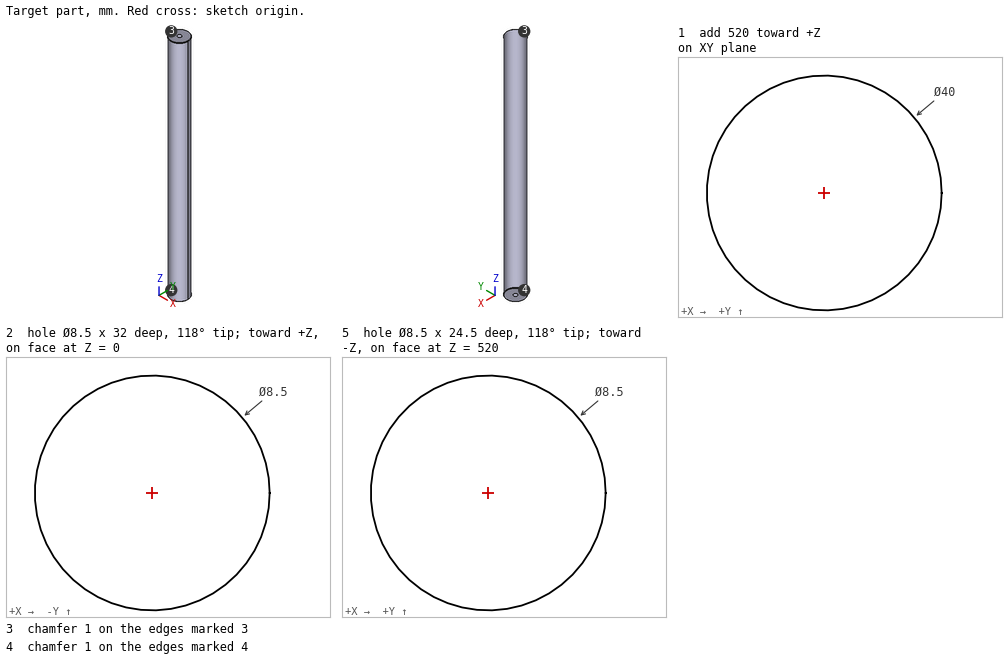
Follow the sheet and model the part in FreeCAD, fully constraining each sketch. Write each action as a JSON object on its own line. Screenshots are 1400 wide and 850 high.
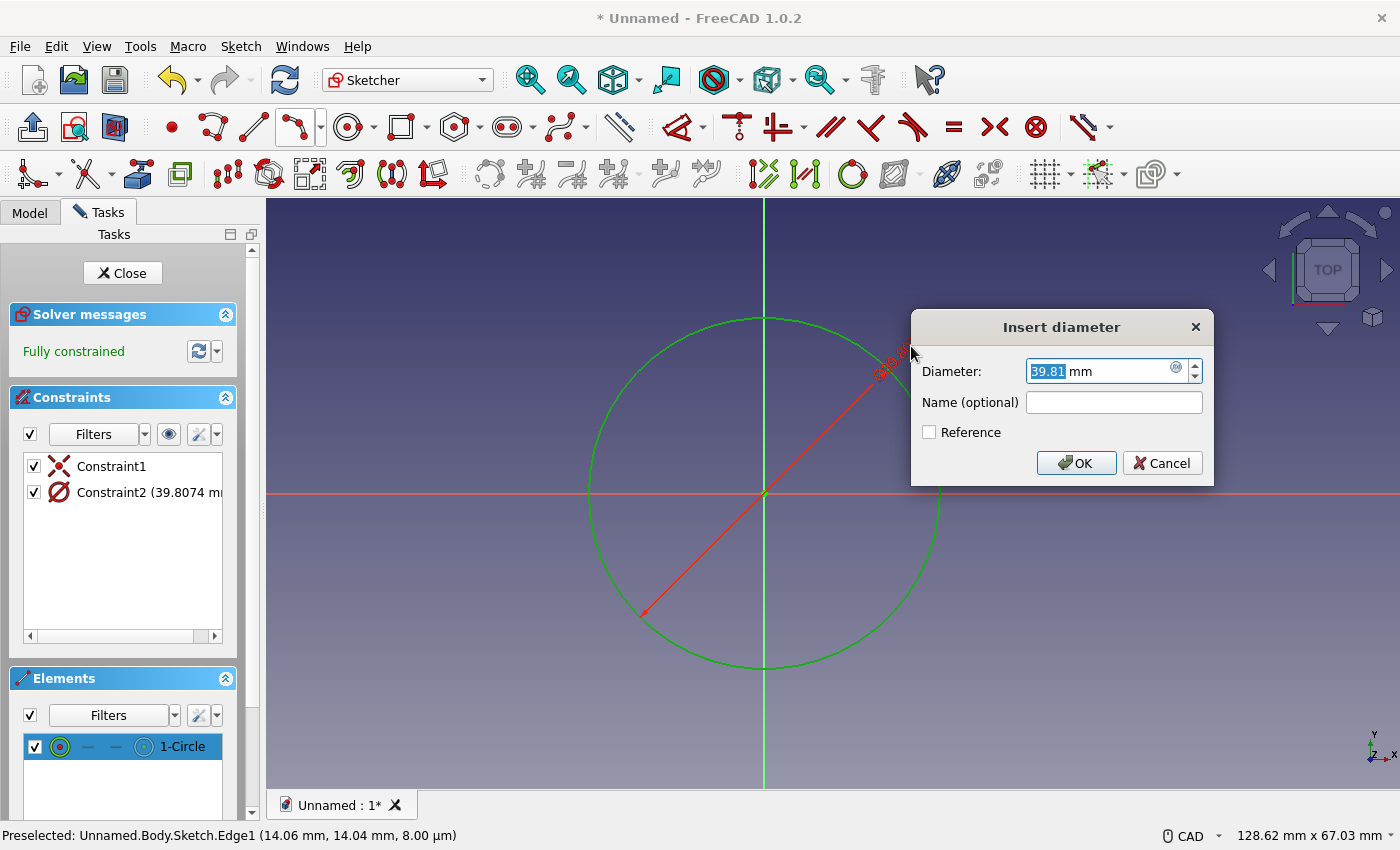
{"action": "type", "text": "40"}
{"action": "key", "text": "Return"}
{"action": "key", "text": "Escape"}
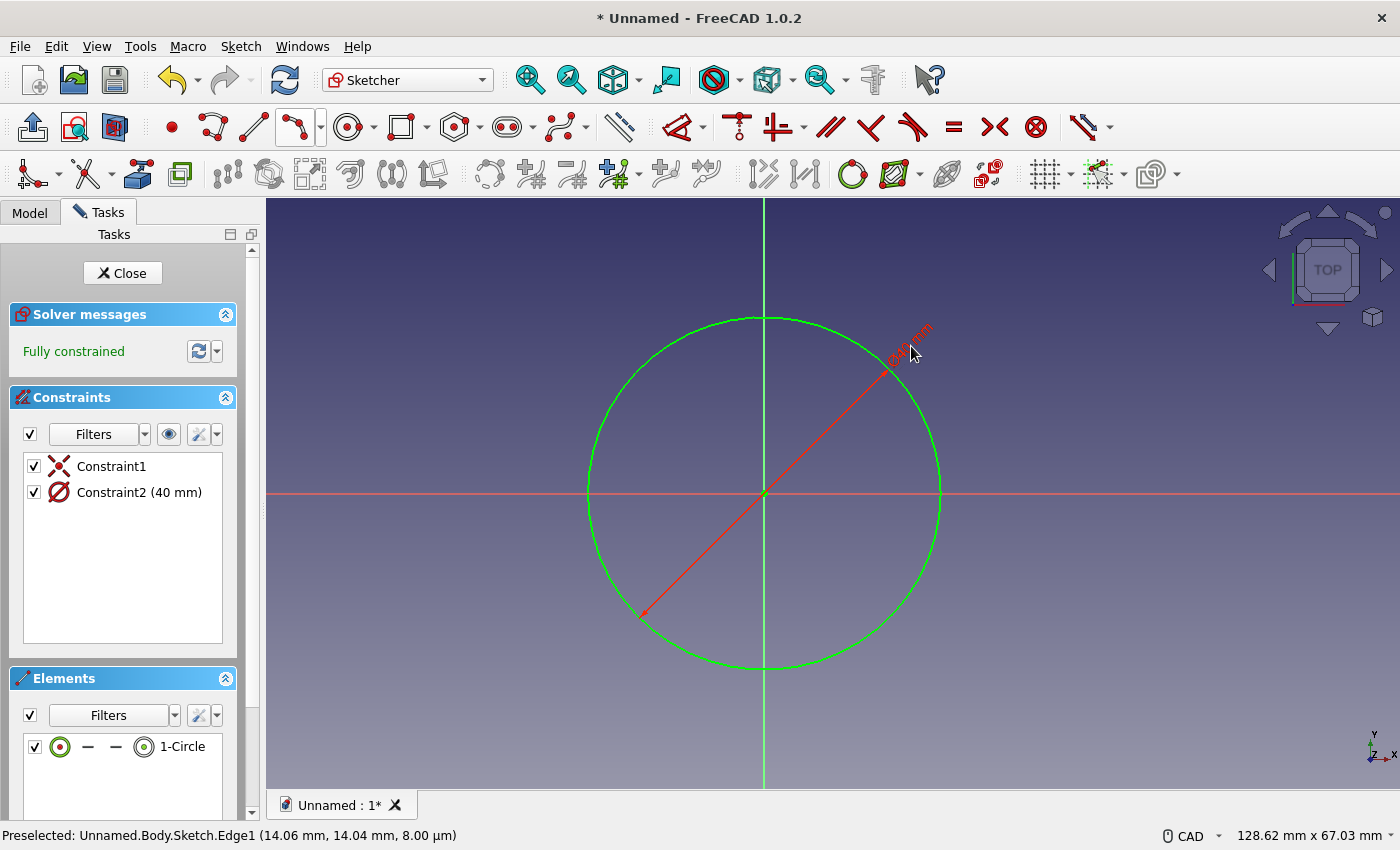
{"action": "left_click", "coordinate": [123, 273]}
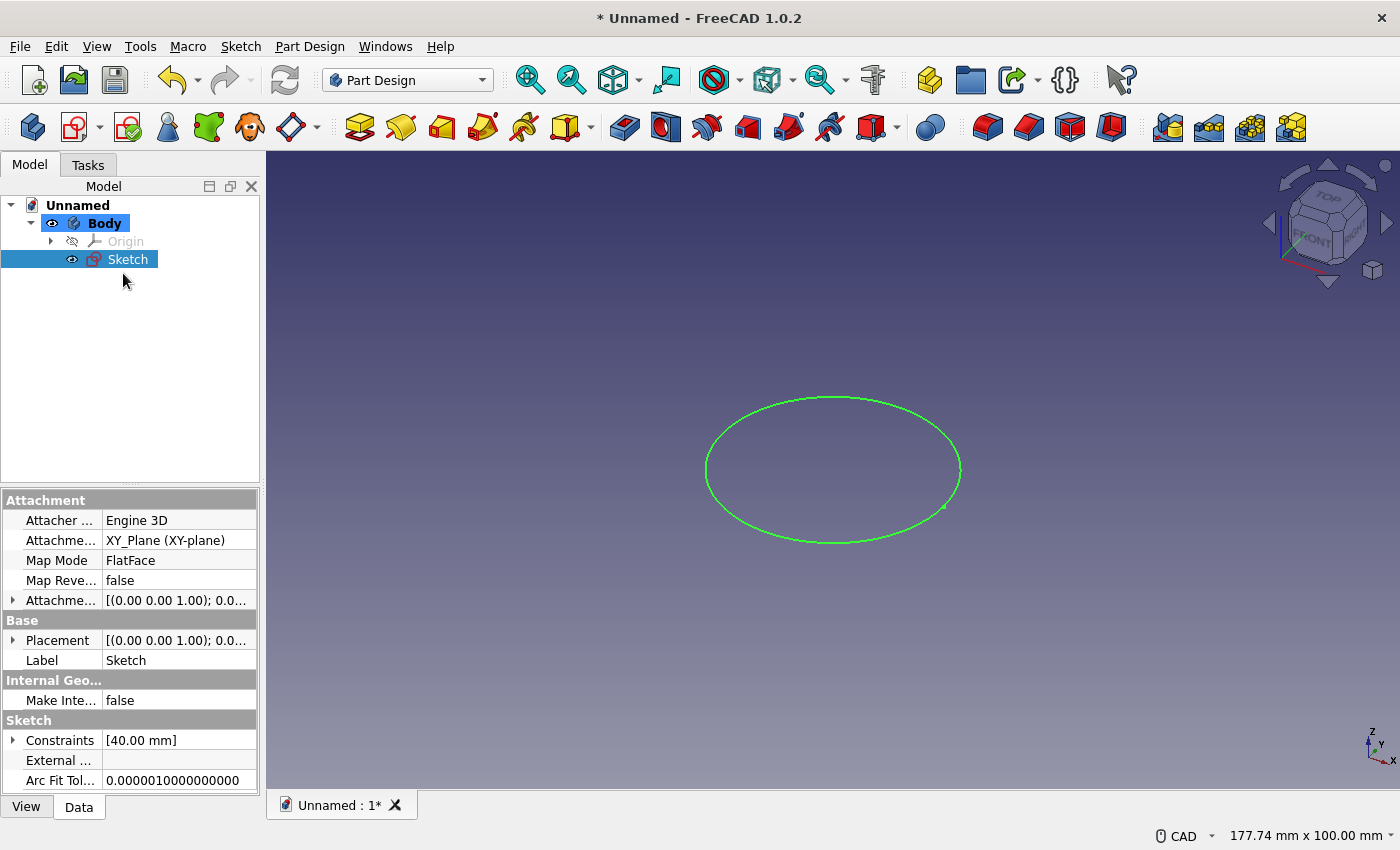
{"action": "left_click", "coordinate": [360, 128]}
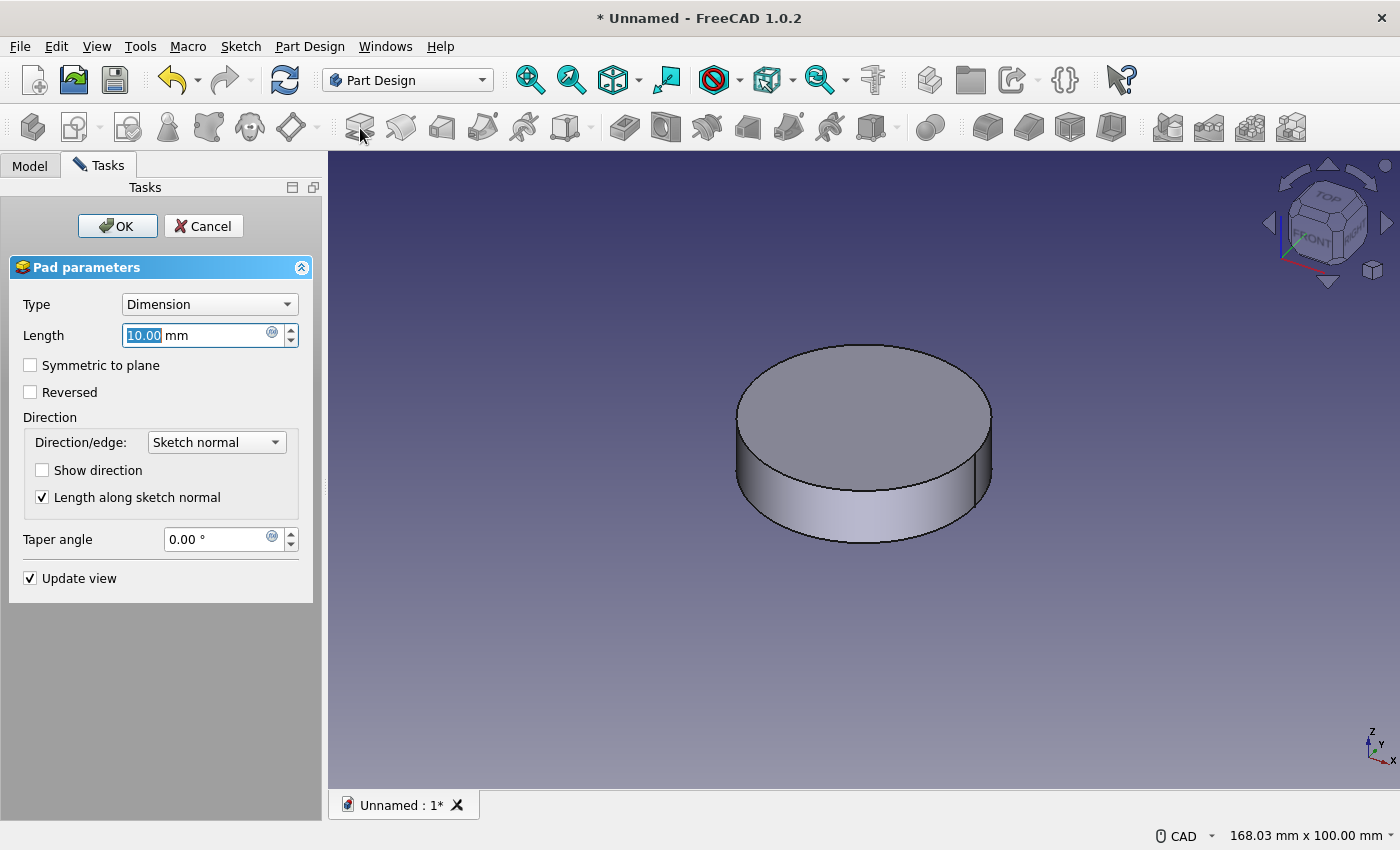
{"action": "type", "text": "520"}
{"action": "key", "text": "Tab"}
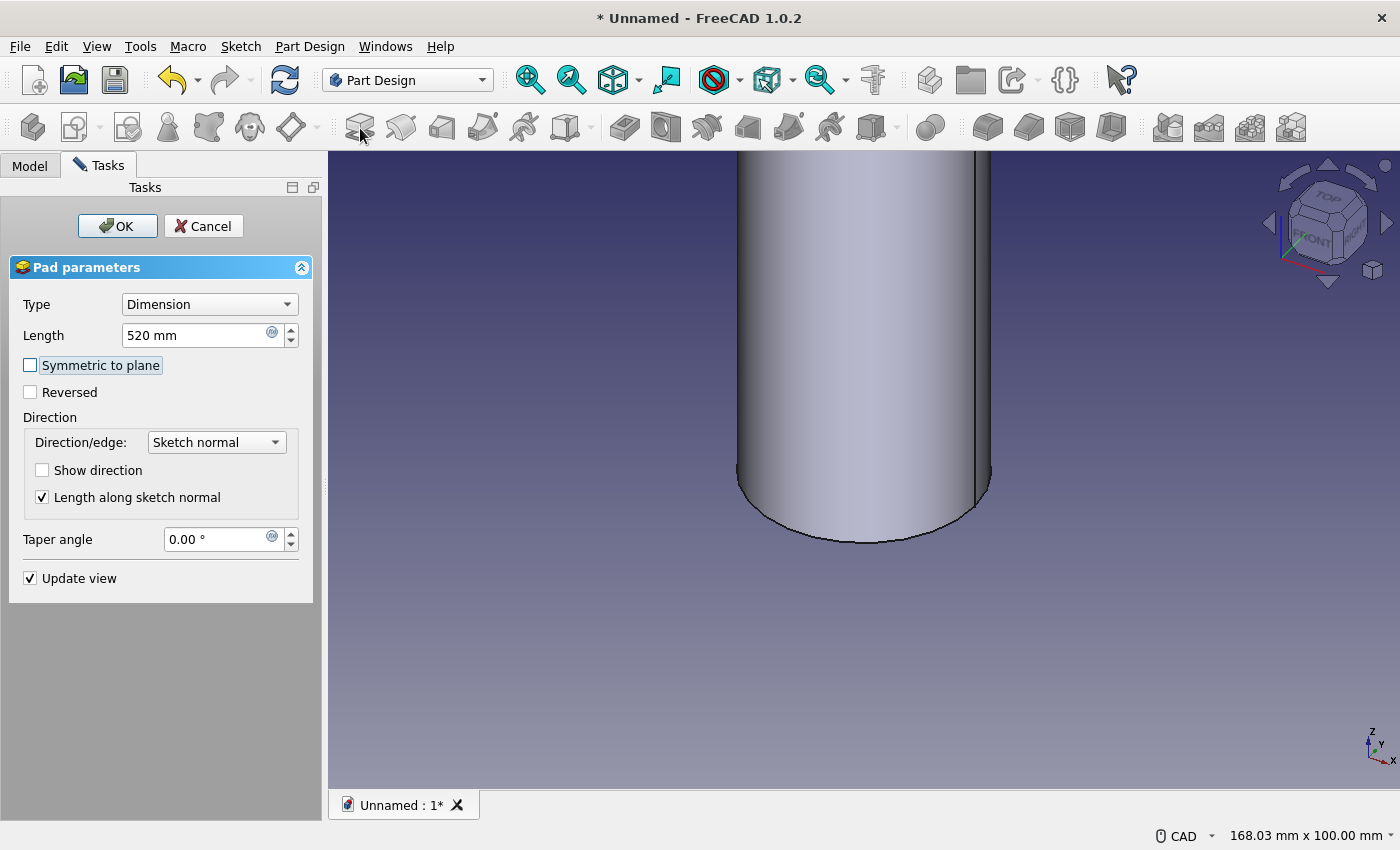
{"action": "left_click", "coordinate": [118, 226]}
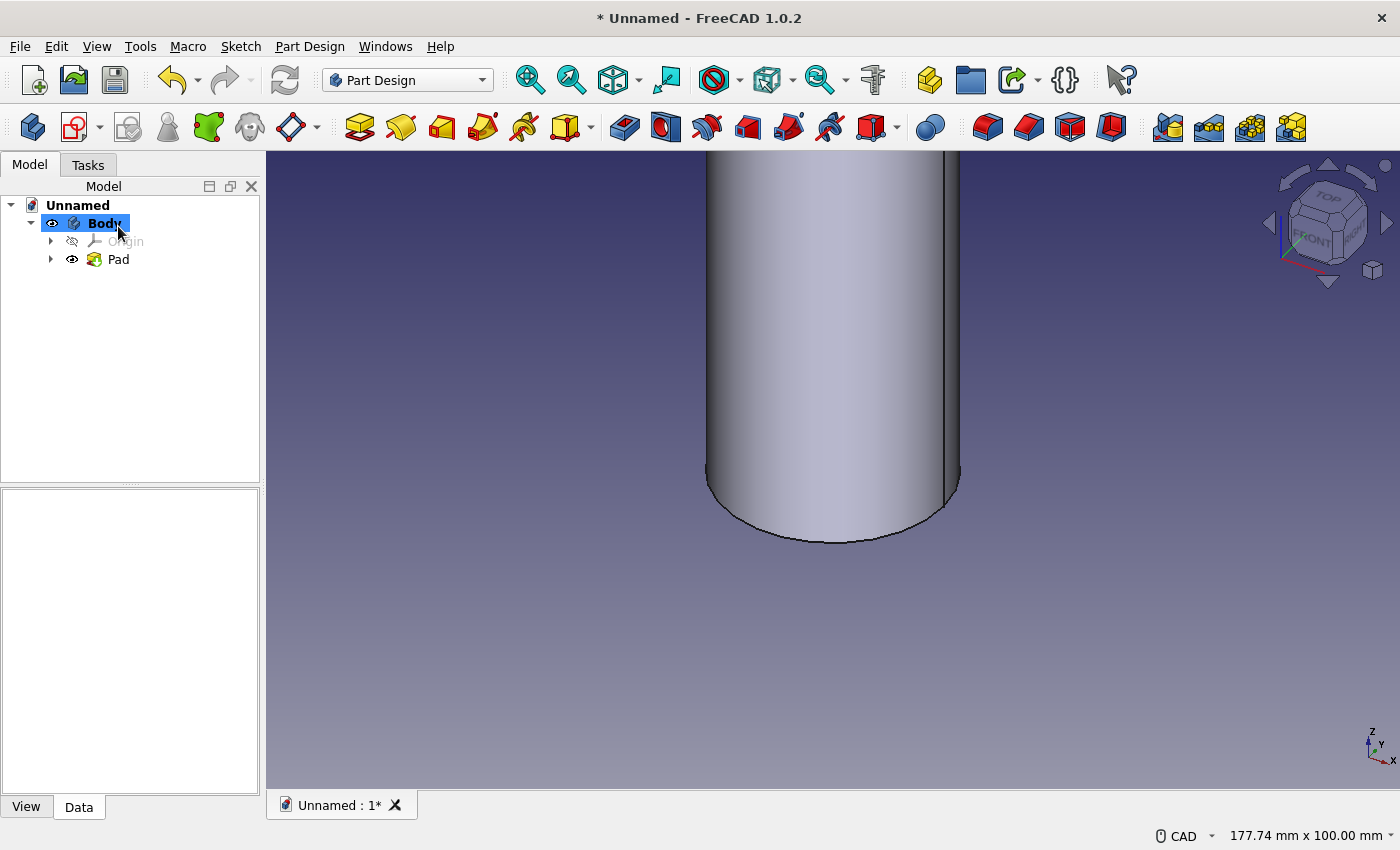
{"action": "left_click", "coordinate": [531, 80]}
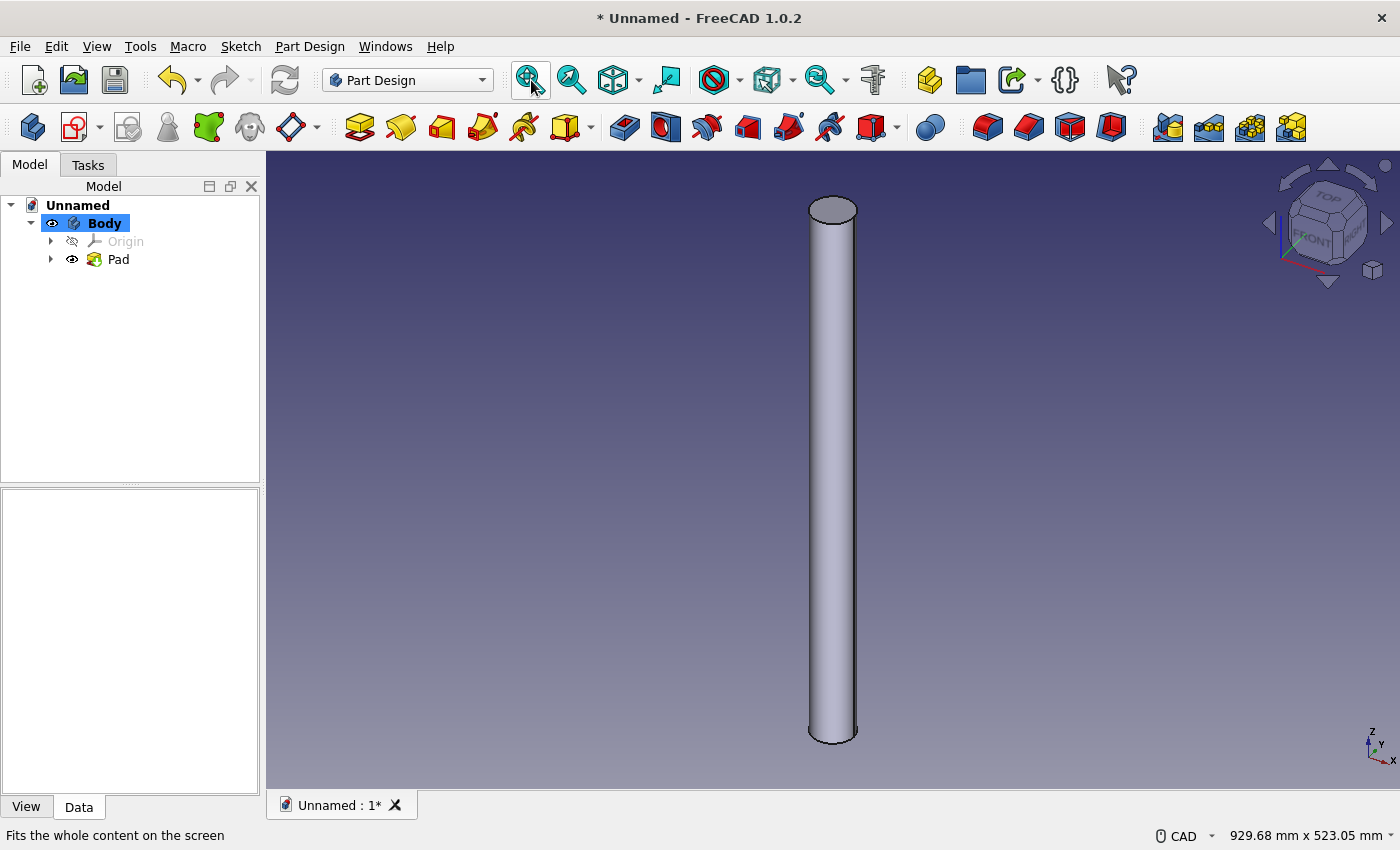
{"action": "key", "text": "5"}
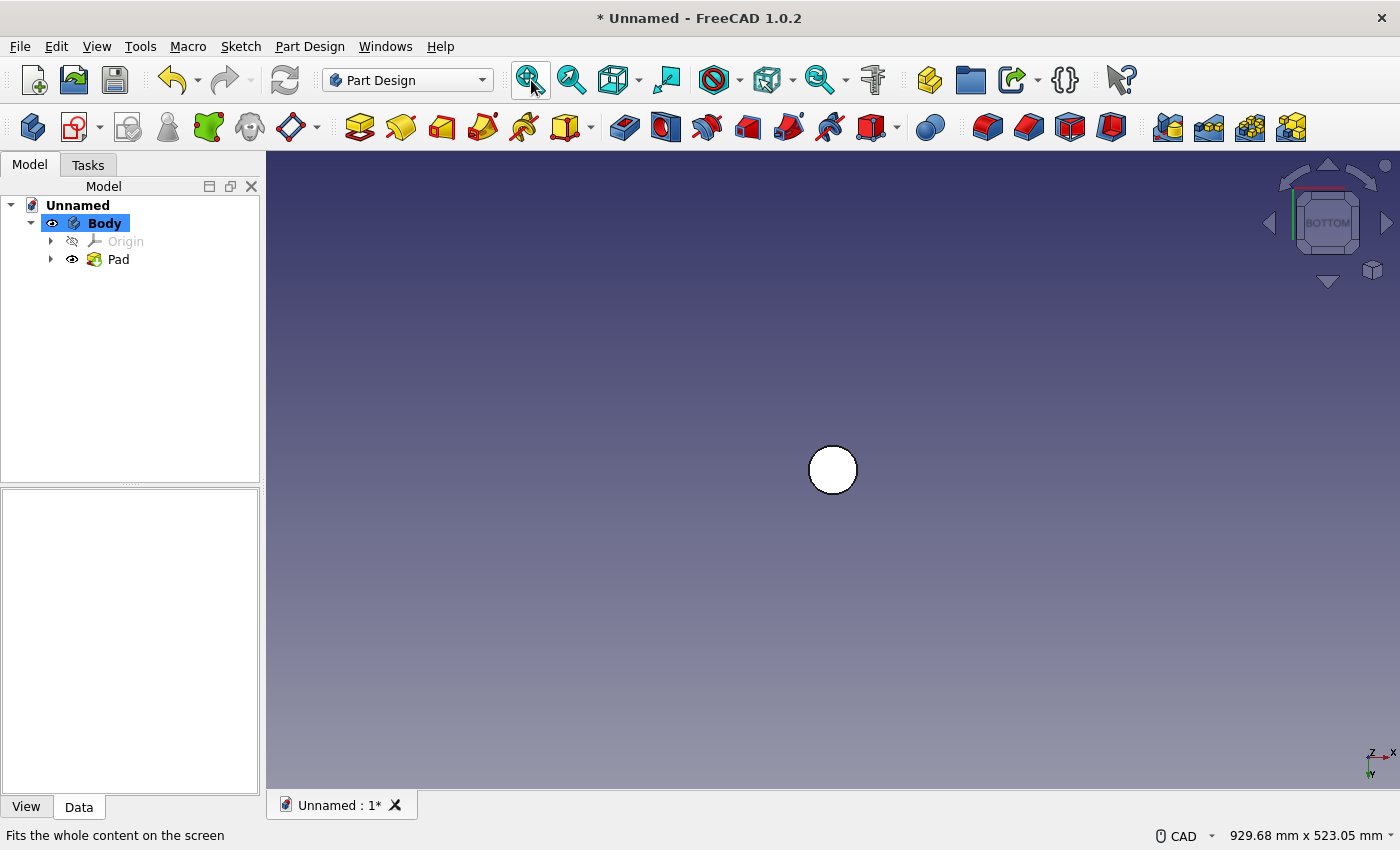
{"action": "left_click", "coordinate": [531, 80]}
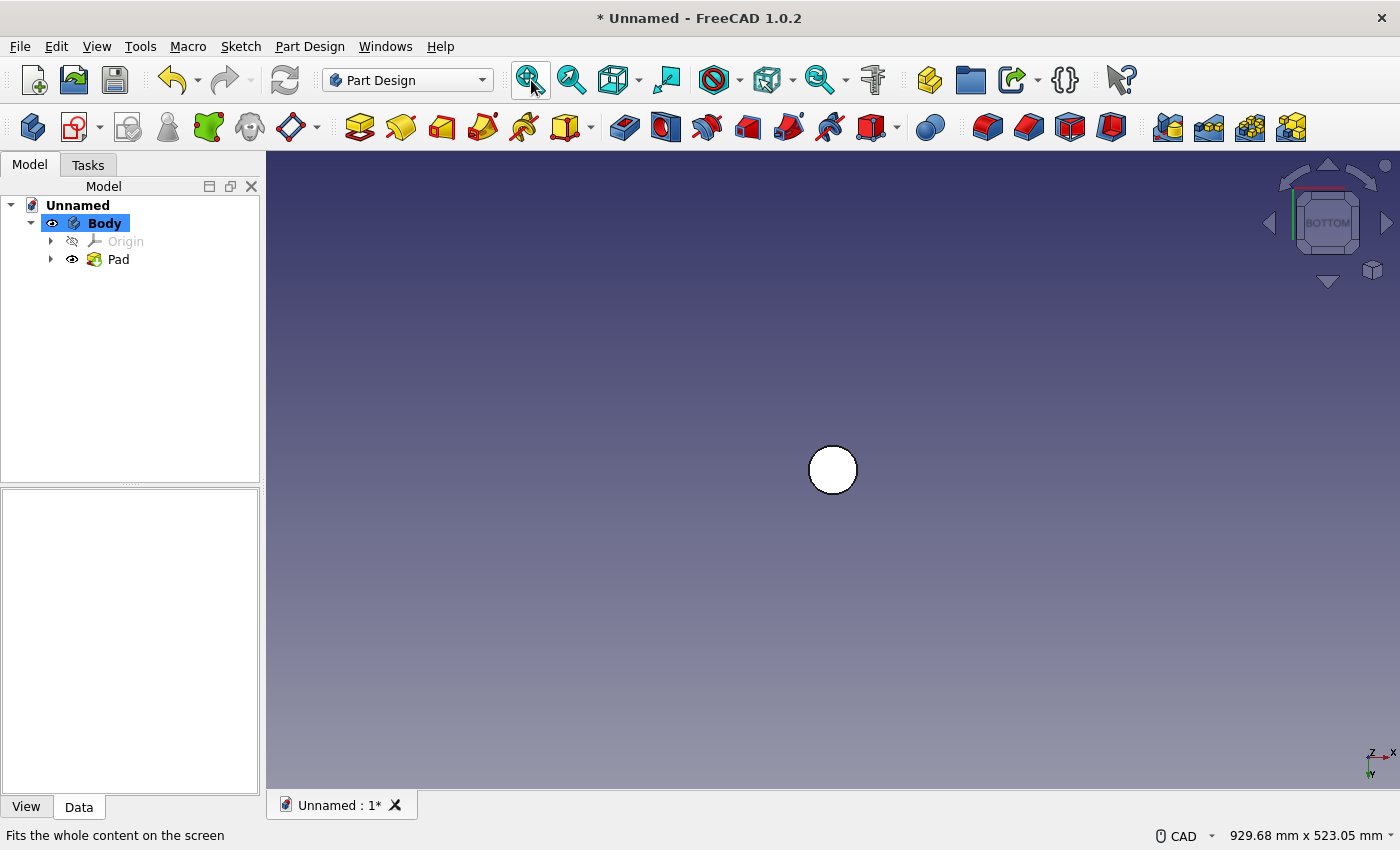
{"action": "left_click", "coordinate": [833, 469]}